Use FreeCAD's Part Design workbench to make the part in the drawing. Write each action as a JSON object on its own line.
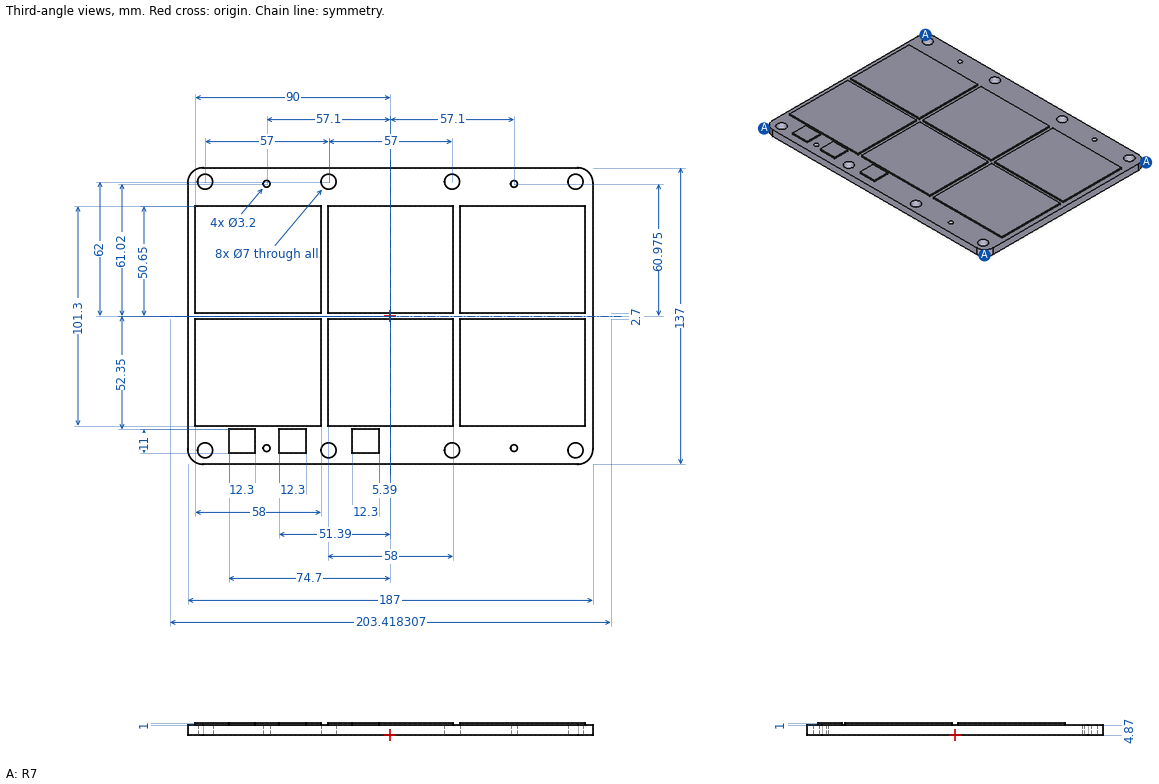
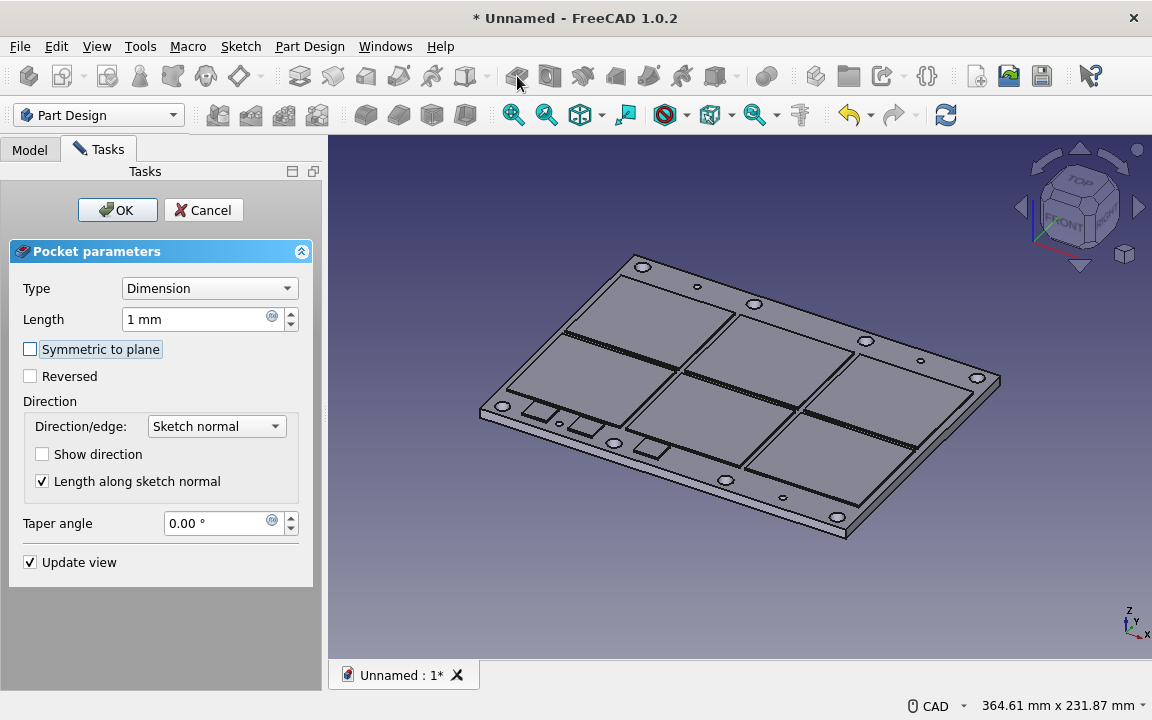
{"action": "left_click", "coordinate": [118, 210]}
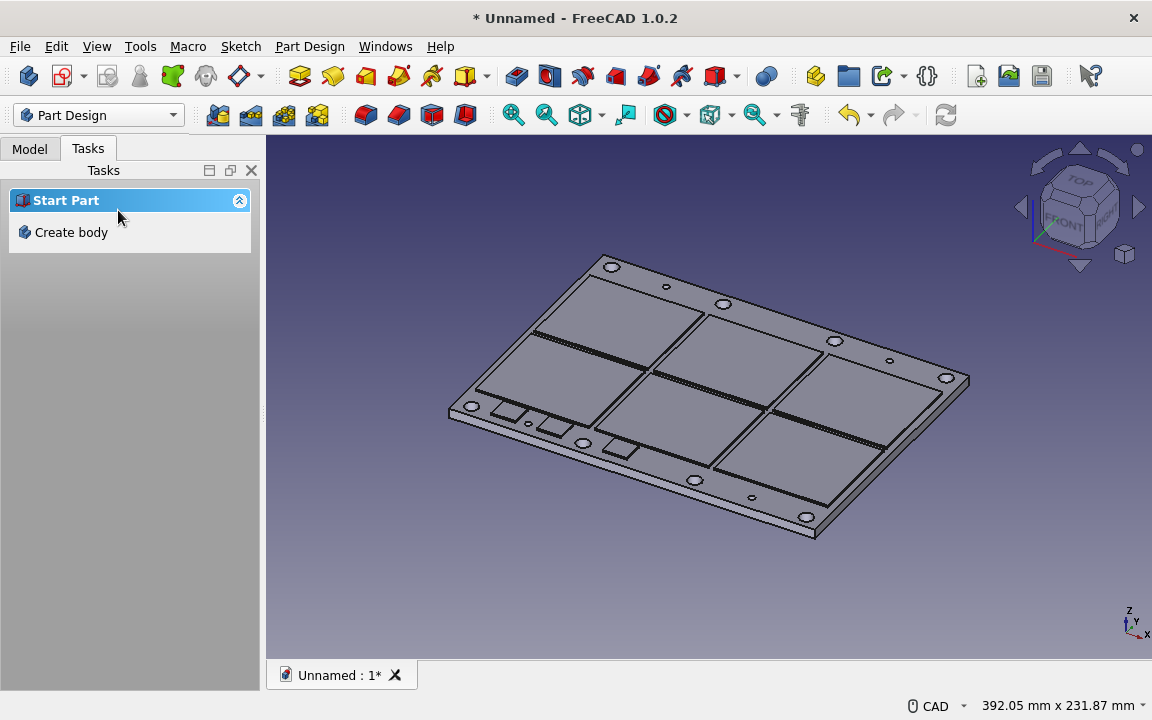
{"action": "left_click", "coordinate": [815, 535]}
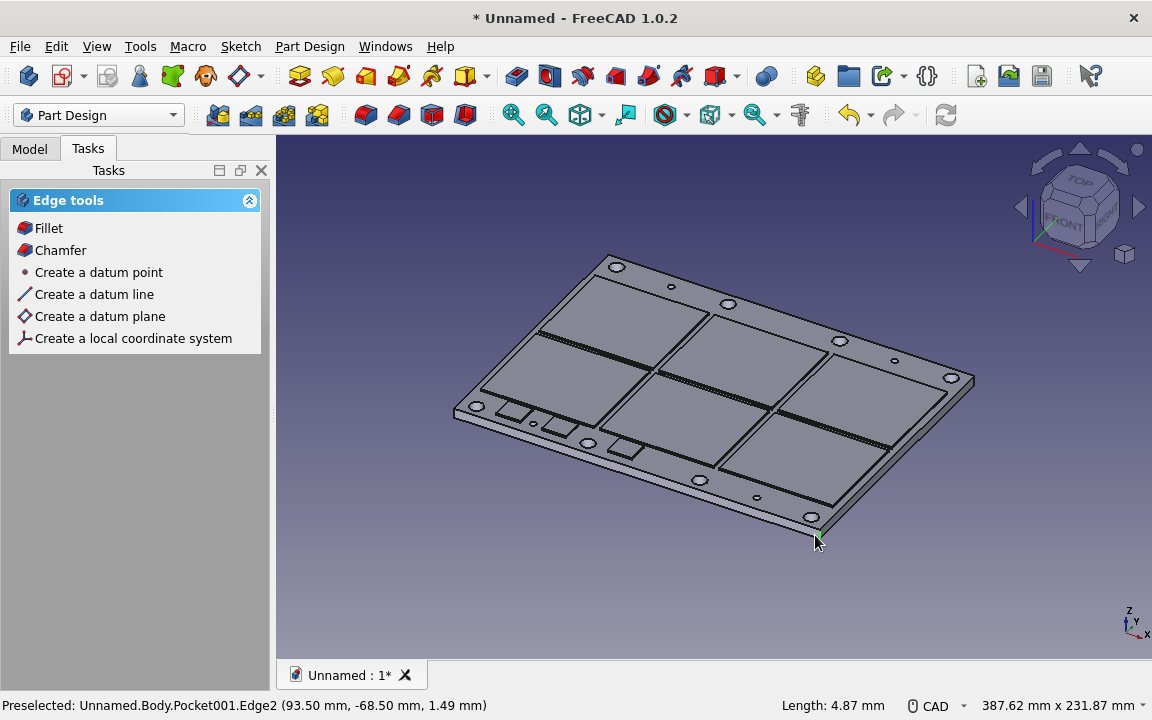
{"action": "scroll", "coordinate": [454, 412], "scroll_direction": "up", "scroll_amount": 7}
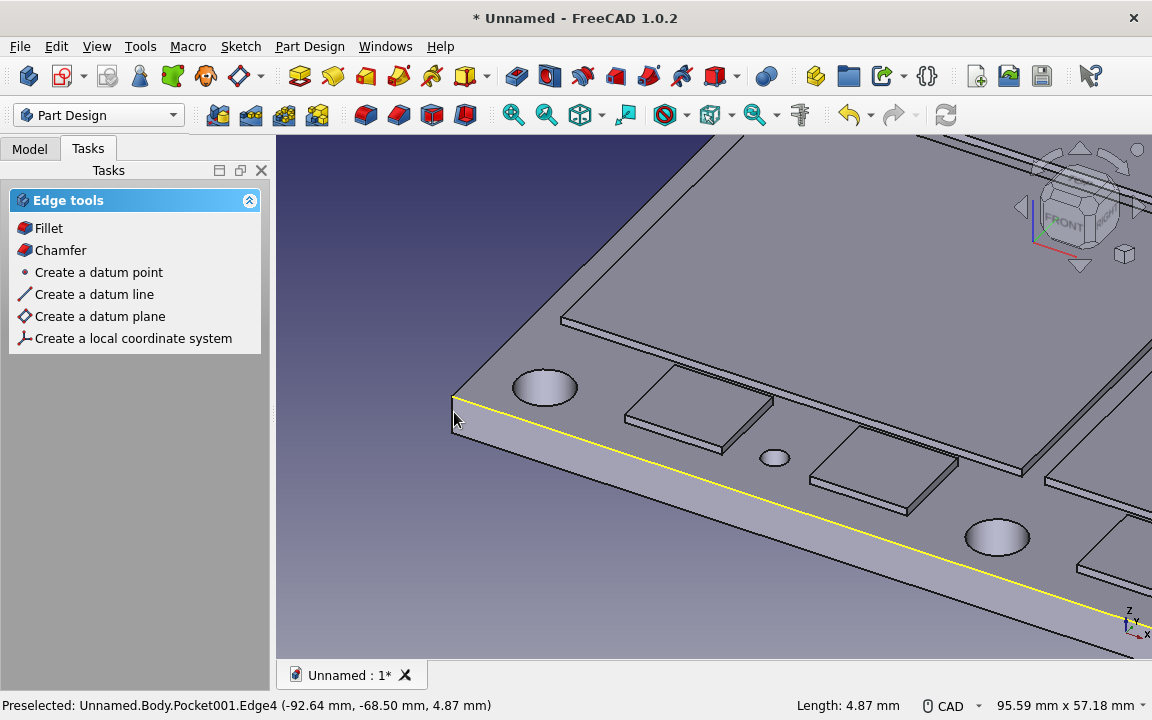
{"action": "key", "text": "v f"}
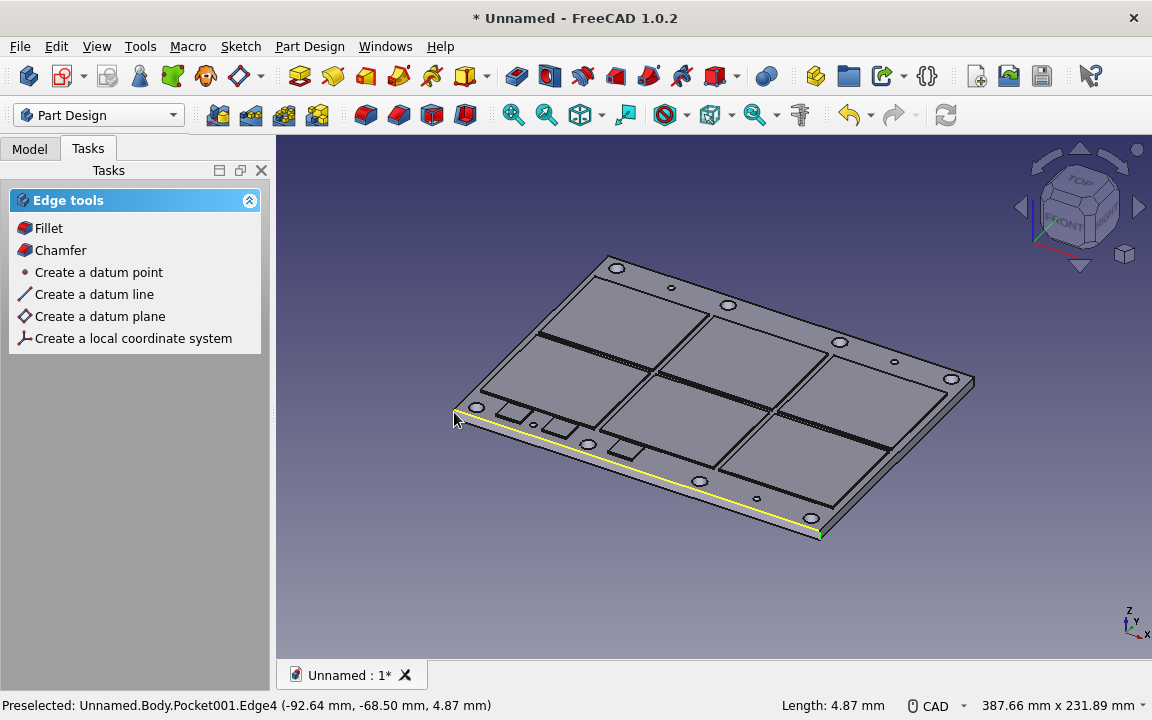
{"action": "key", "text": "0"}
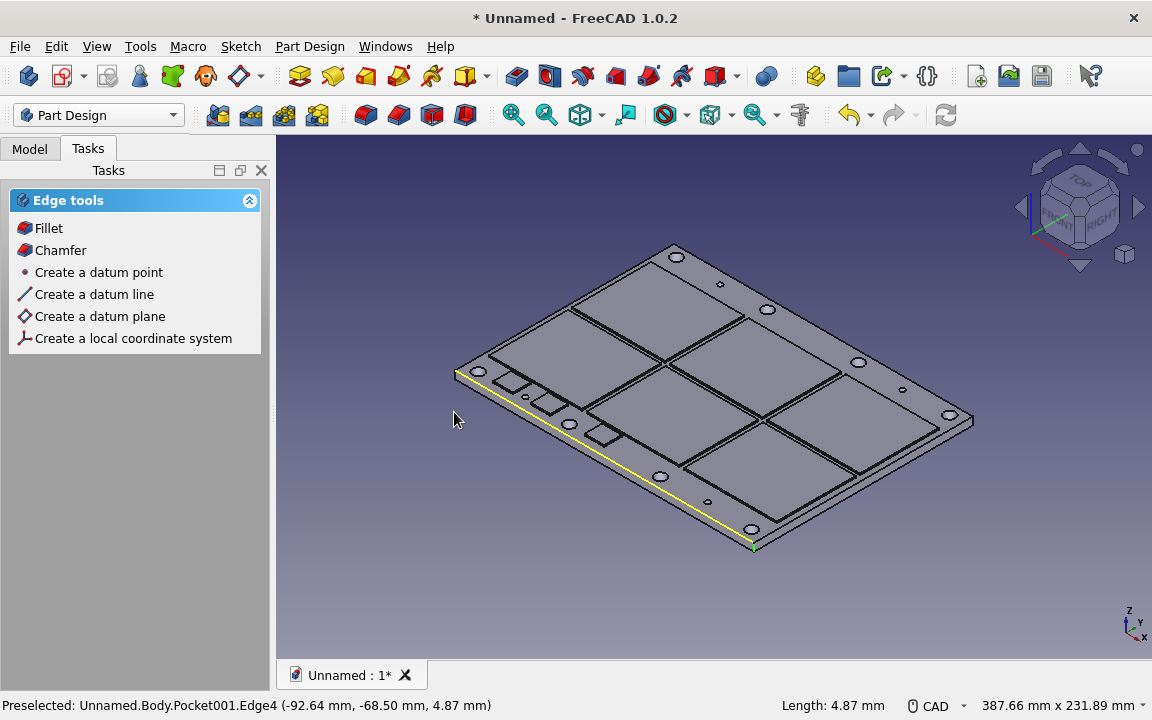
{"action": "scroll", "coordinate": [455, 374], "scroll_direction": "up", "scroll_amount": 7}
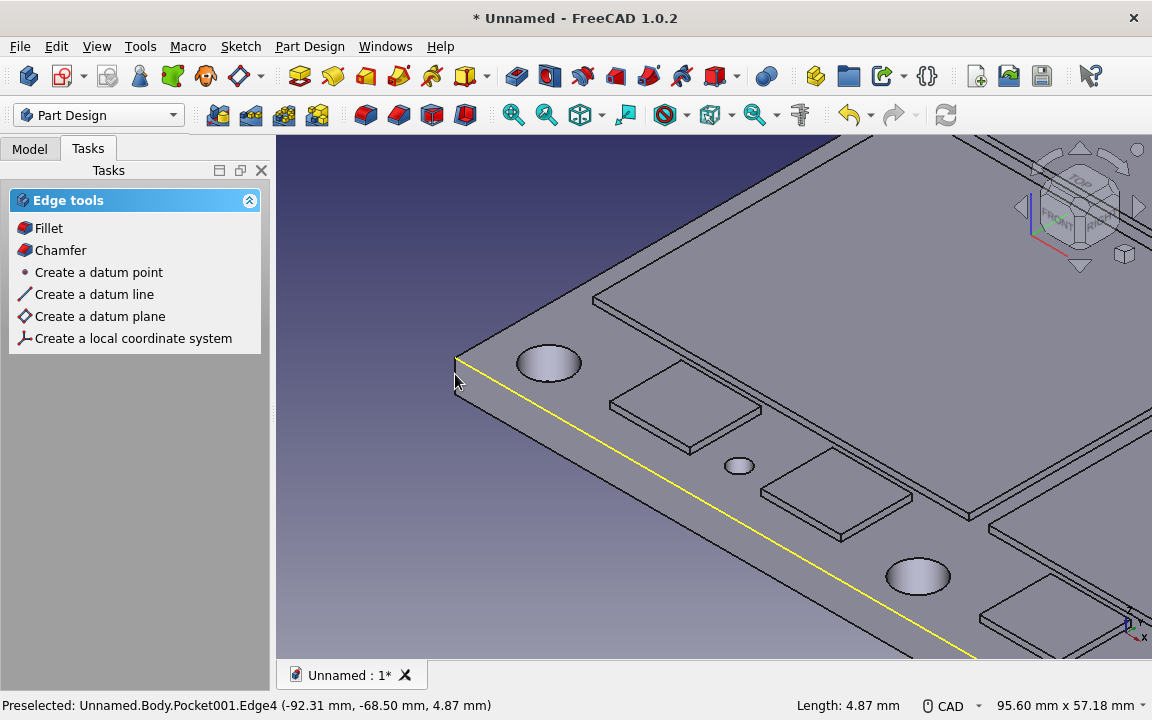
{"action": "key", "text": "v f"}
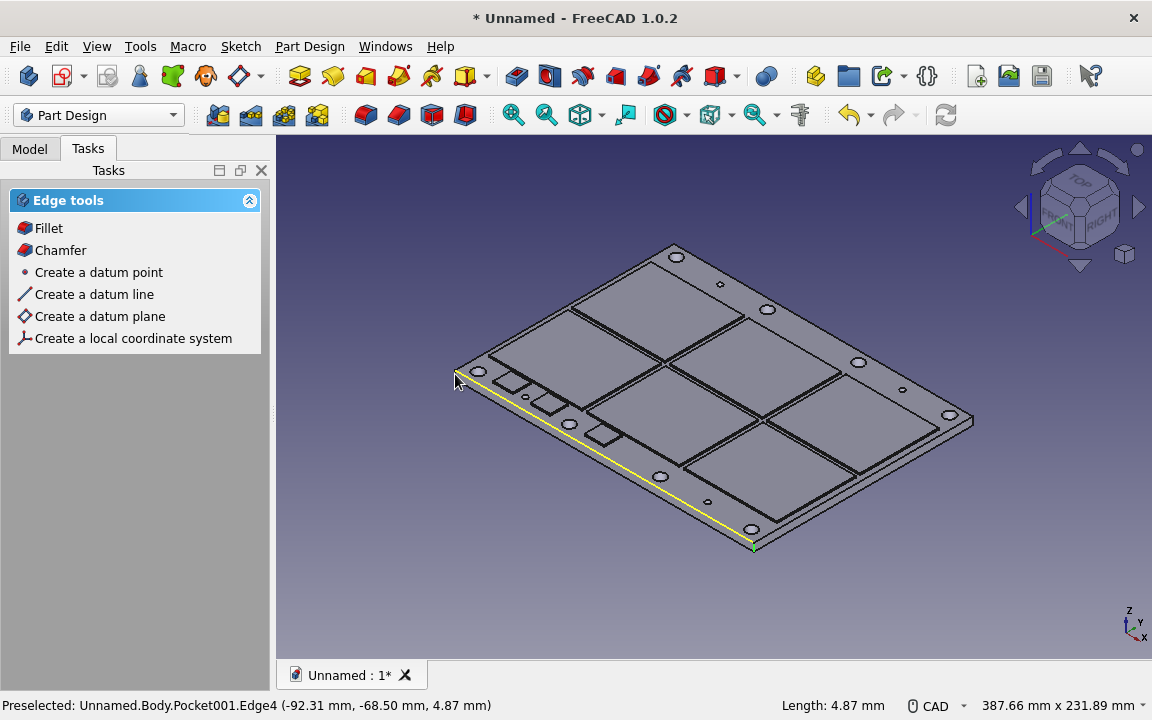
{"action": "key", "text": "2"}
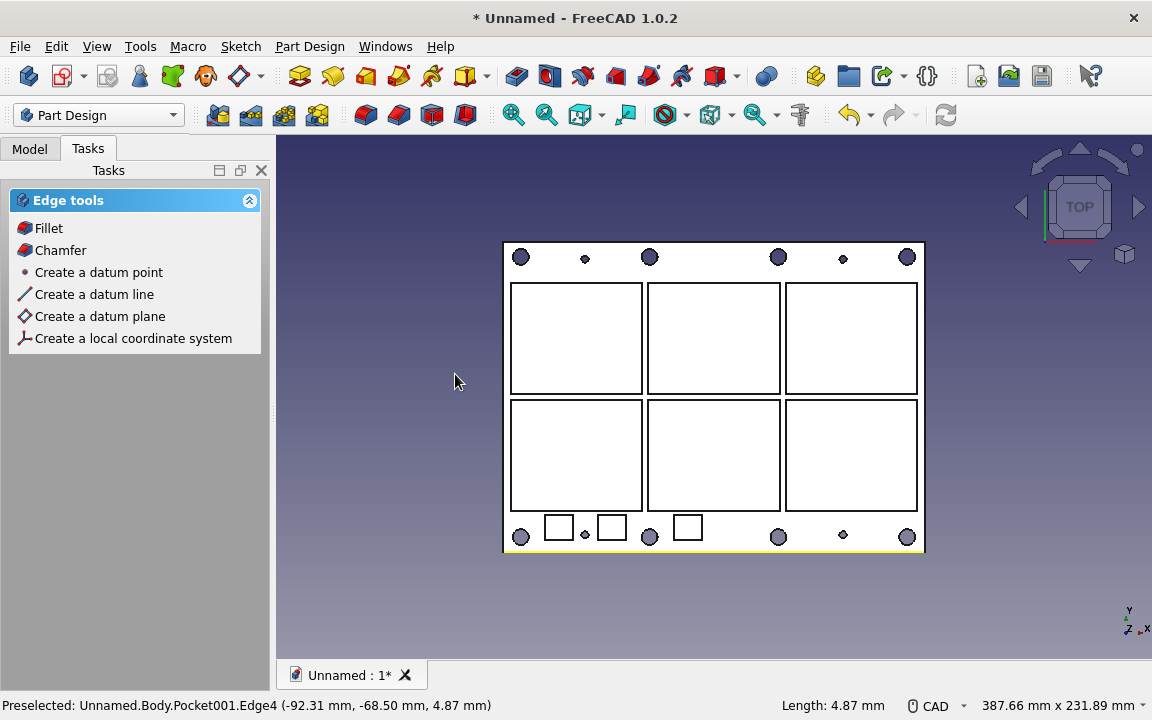
{"action": "scroll", "coordinate": [503, 551], "scroll_direction": "up", "scroll_amount": 7}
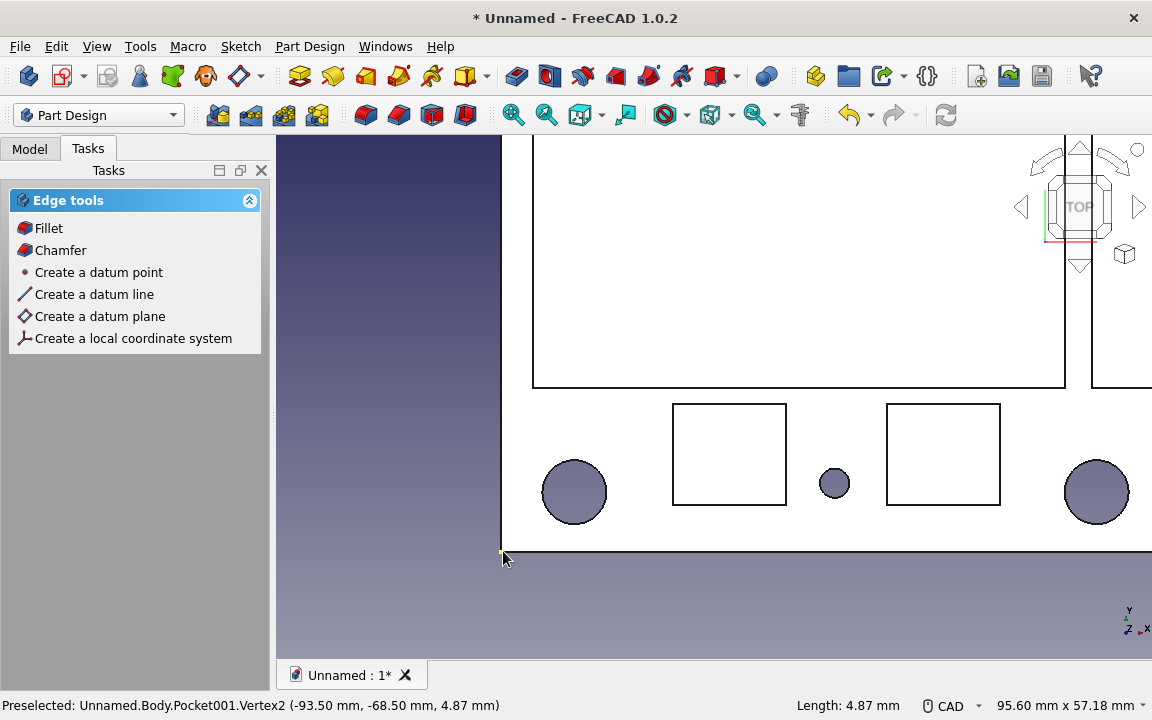
{"action": "key", "text": "v f"}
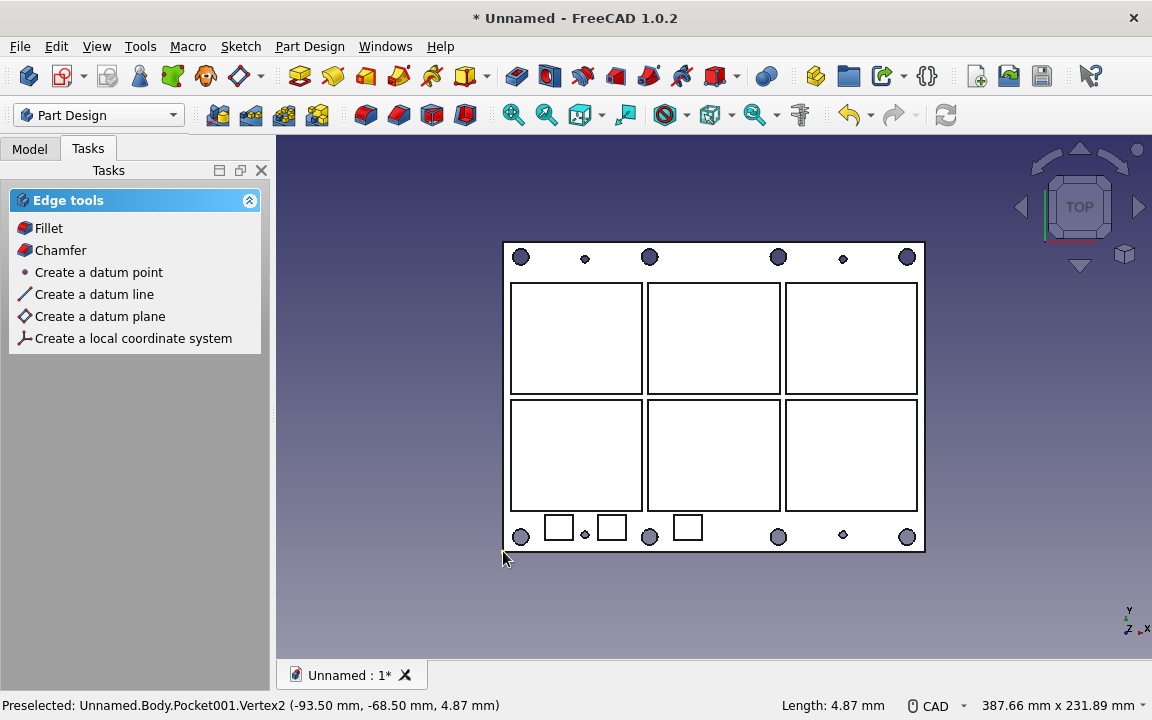
{"action": "key", "text": "1"}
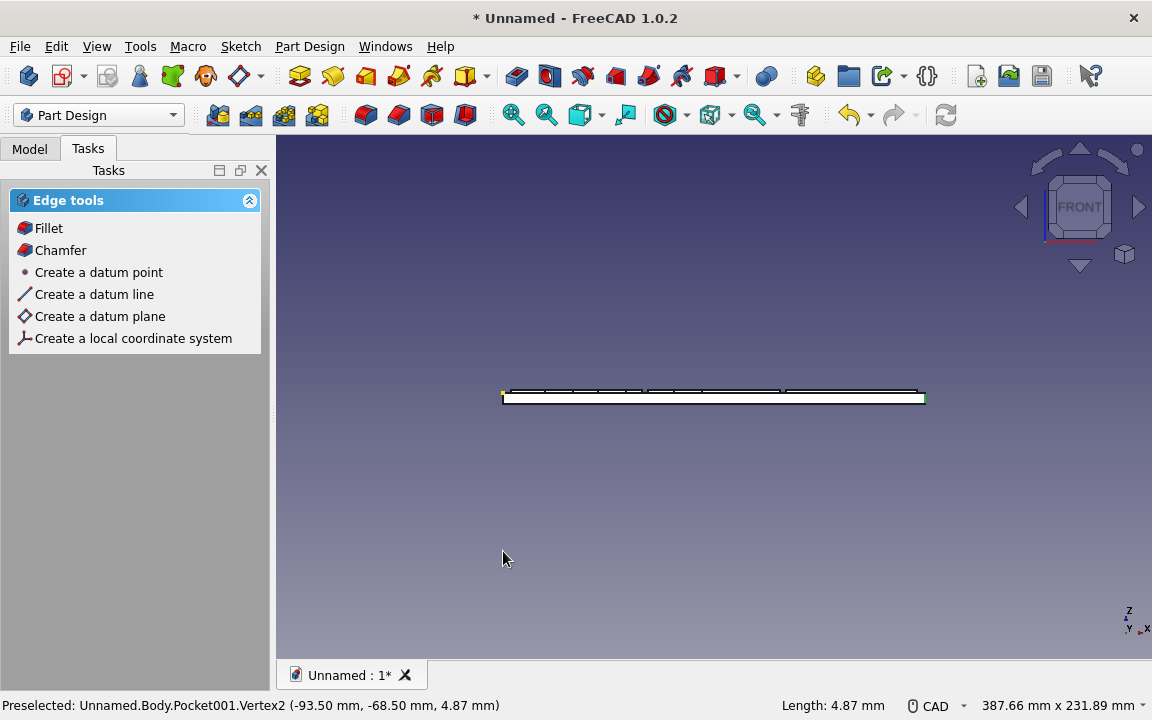
{"action": "scroll", "coordinate": [503, 397], "scroll_direction": "up", "scroll_amount": 7}